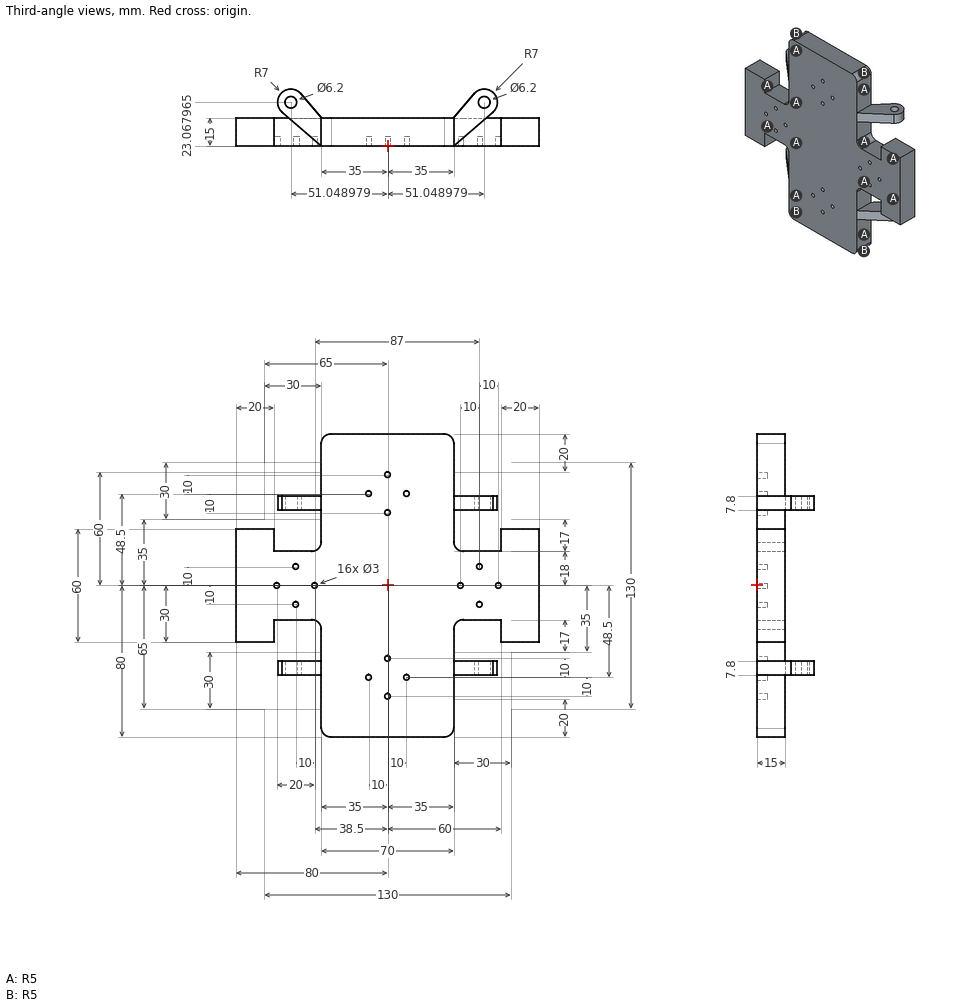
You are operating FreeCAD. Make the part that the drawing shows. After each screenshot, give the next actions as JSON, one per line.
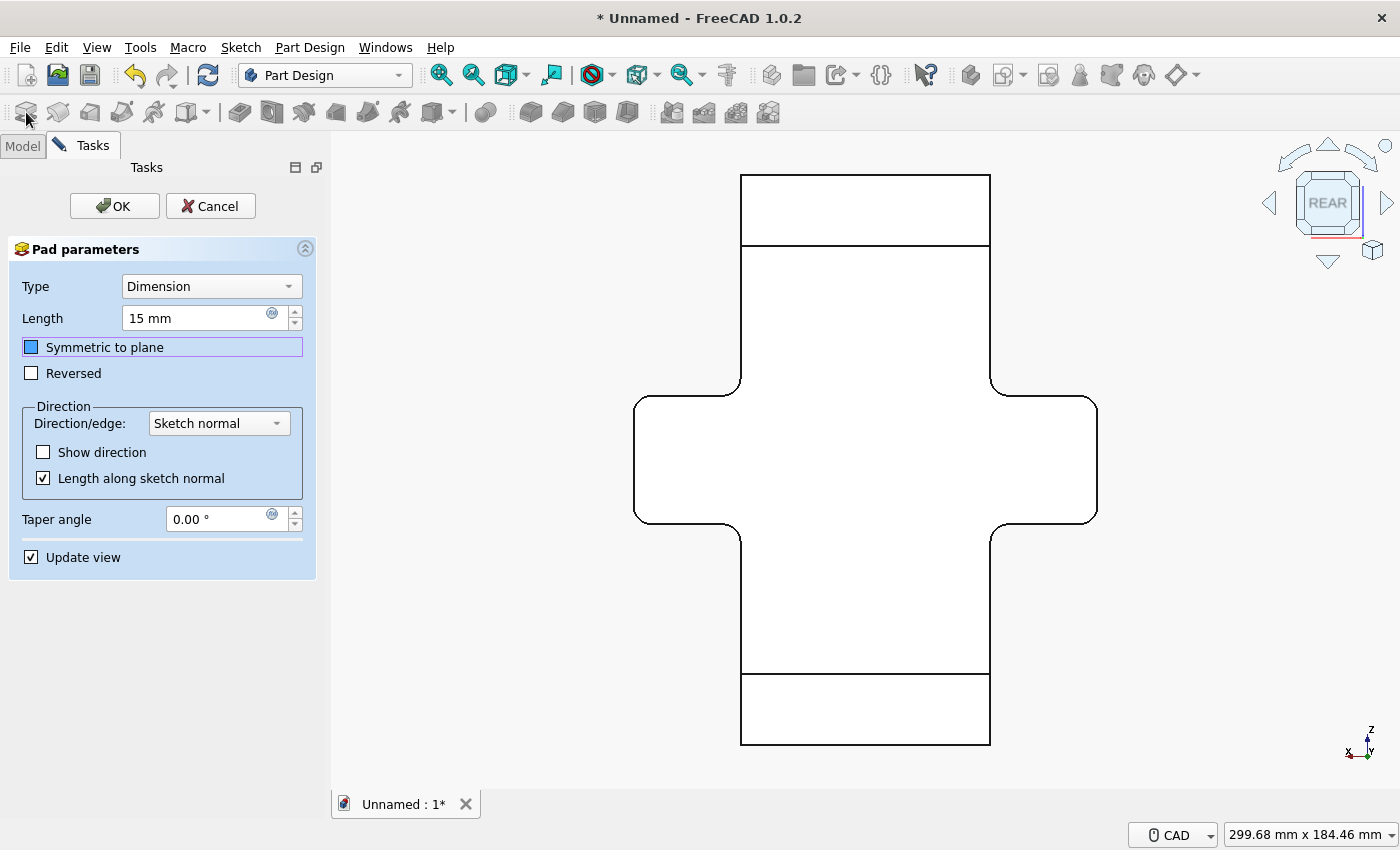
{"action": "left_click", "coordinate": [30, 373]}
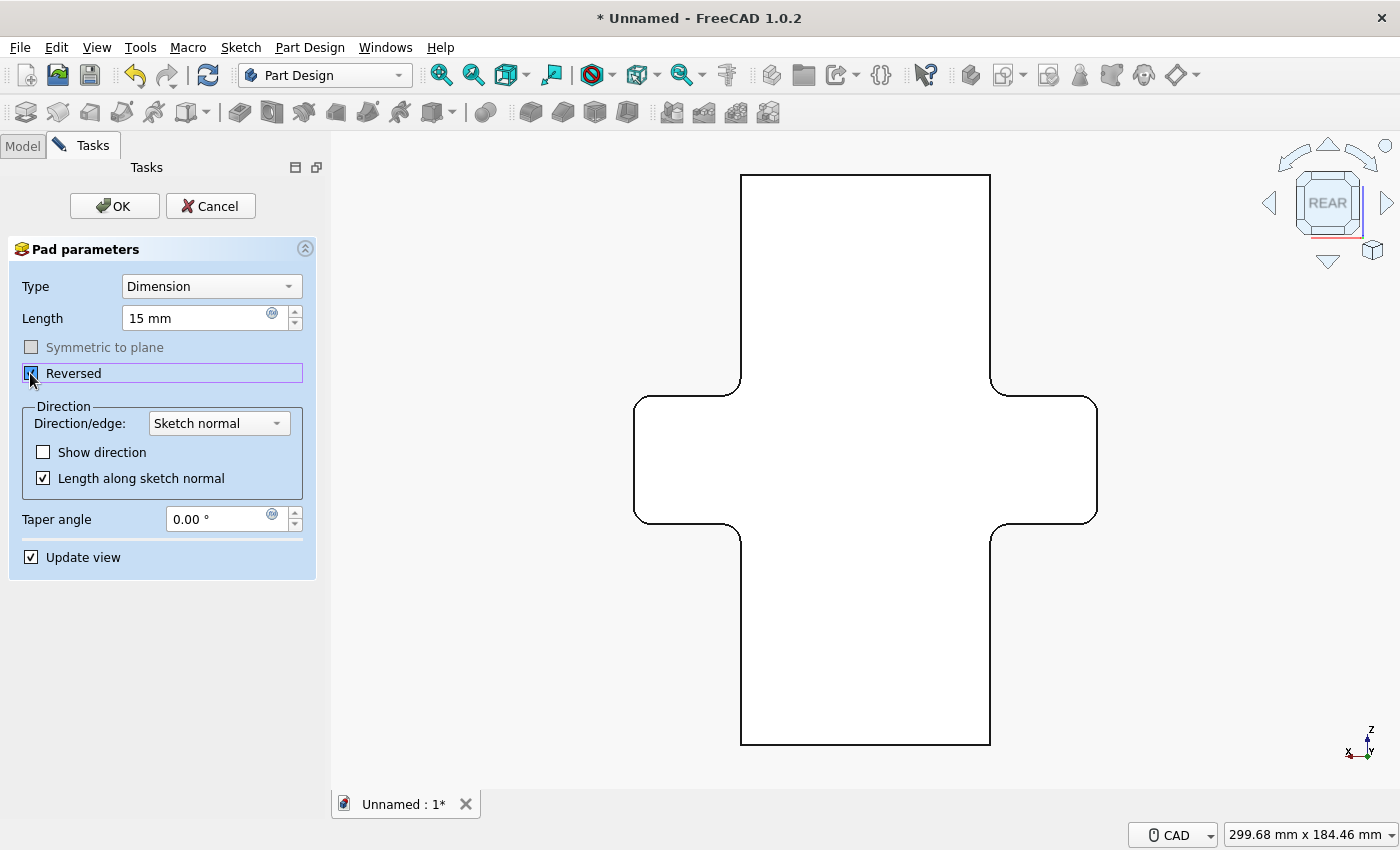
{"action": "left_click", "coordinate": [115, 206]}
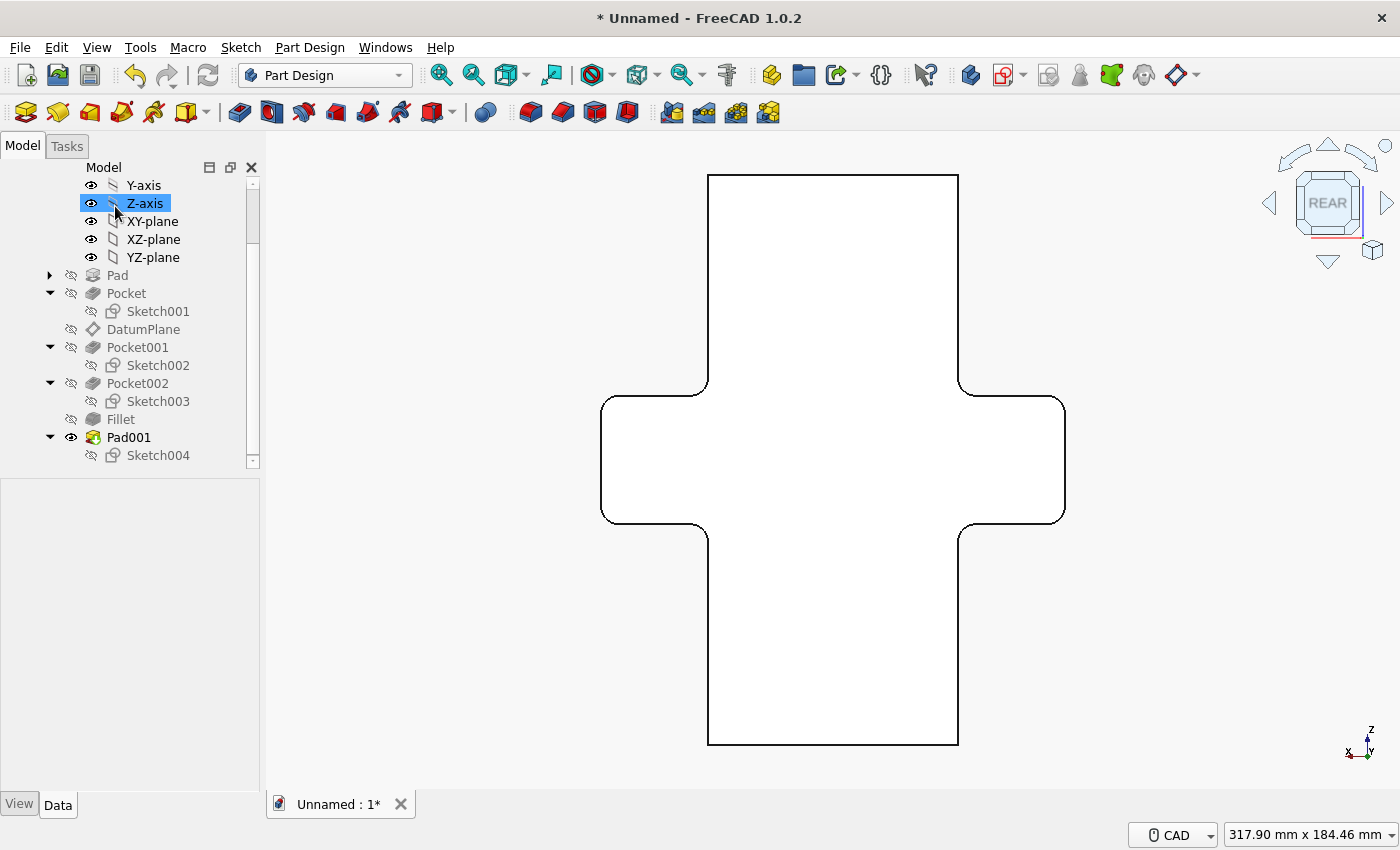
{"action": "scroll", "coordinate": [160, 325], "scroll_direction": "down", "scroll_amount": 3}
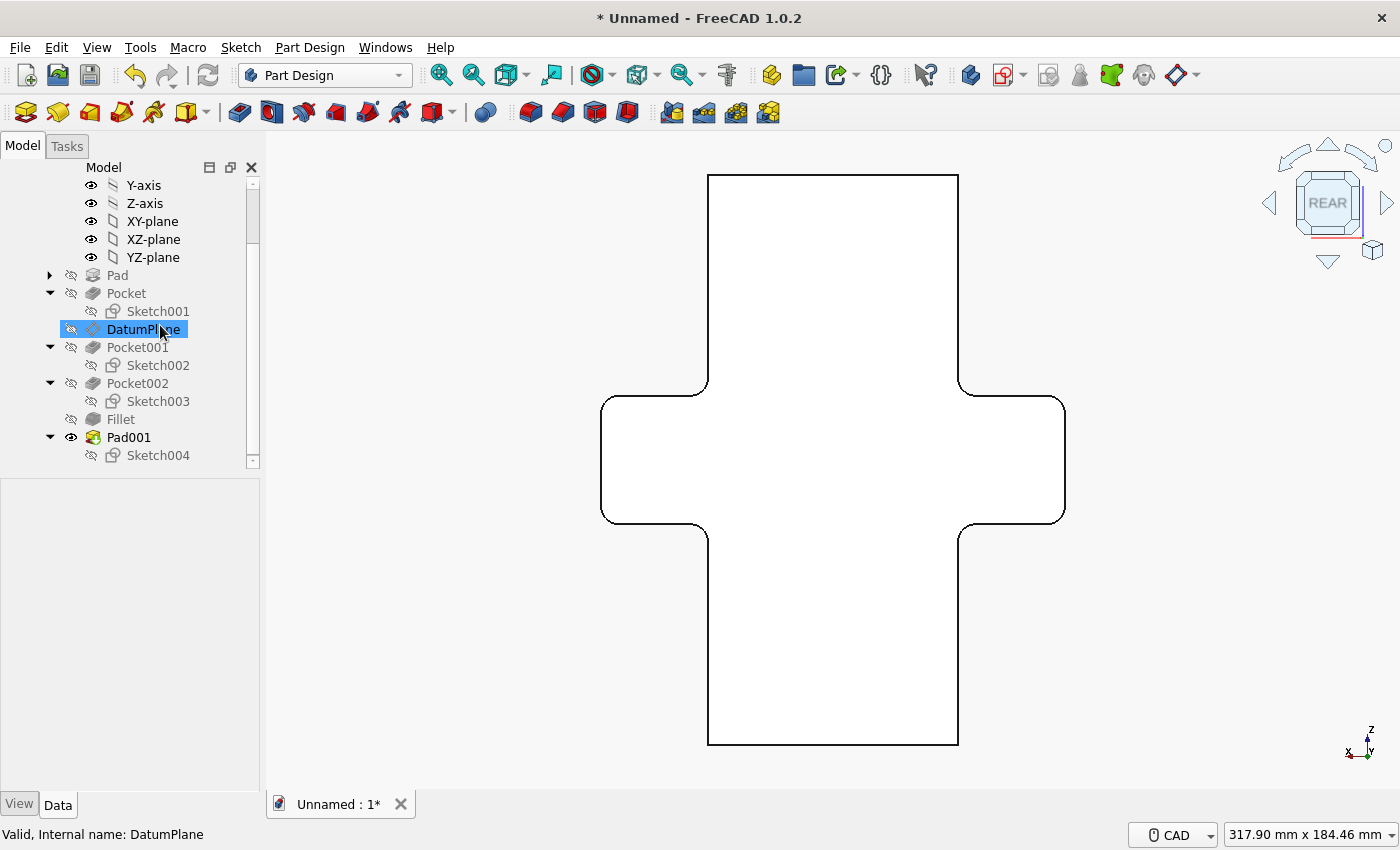
{"action": "scroll", "coordinate": [160, 325], "scroll_direction": "up", "scroll_amount": 15}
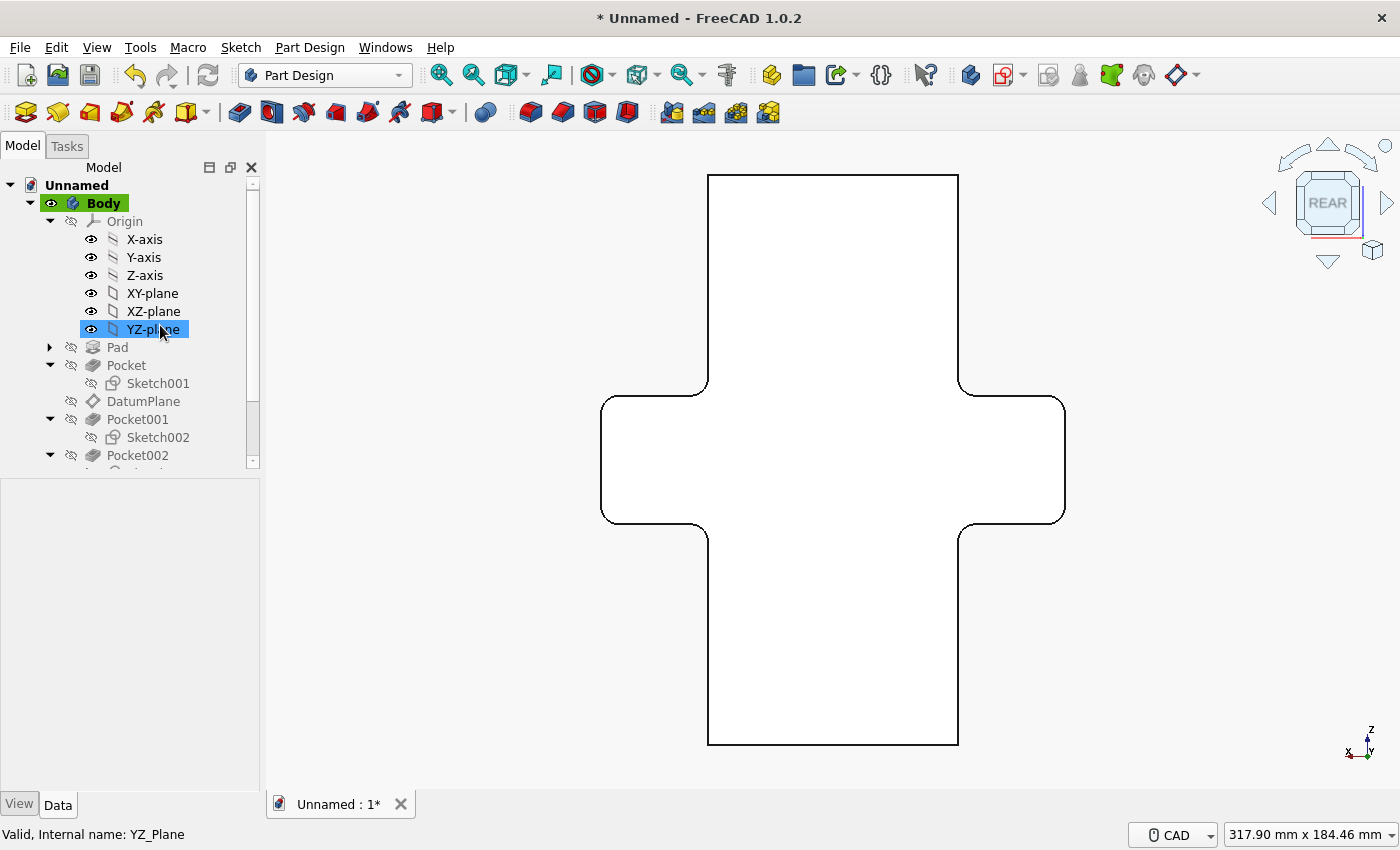
{"action": "left_click", "coordinate": [136, 293]}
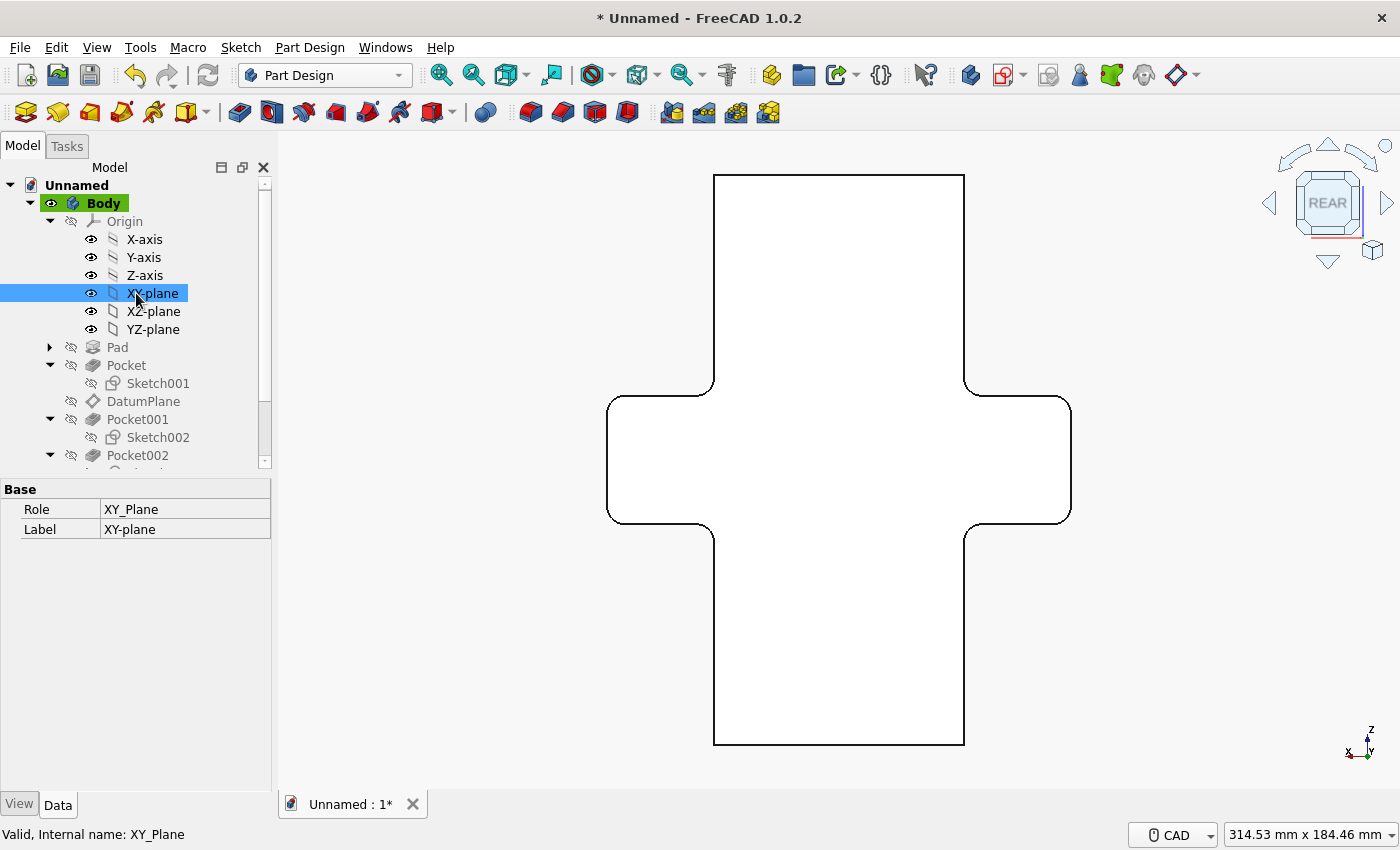
{"action": "left_click", "coordinate": [1176, 76]}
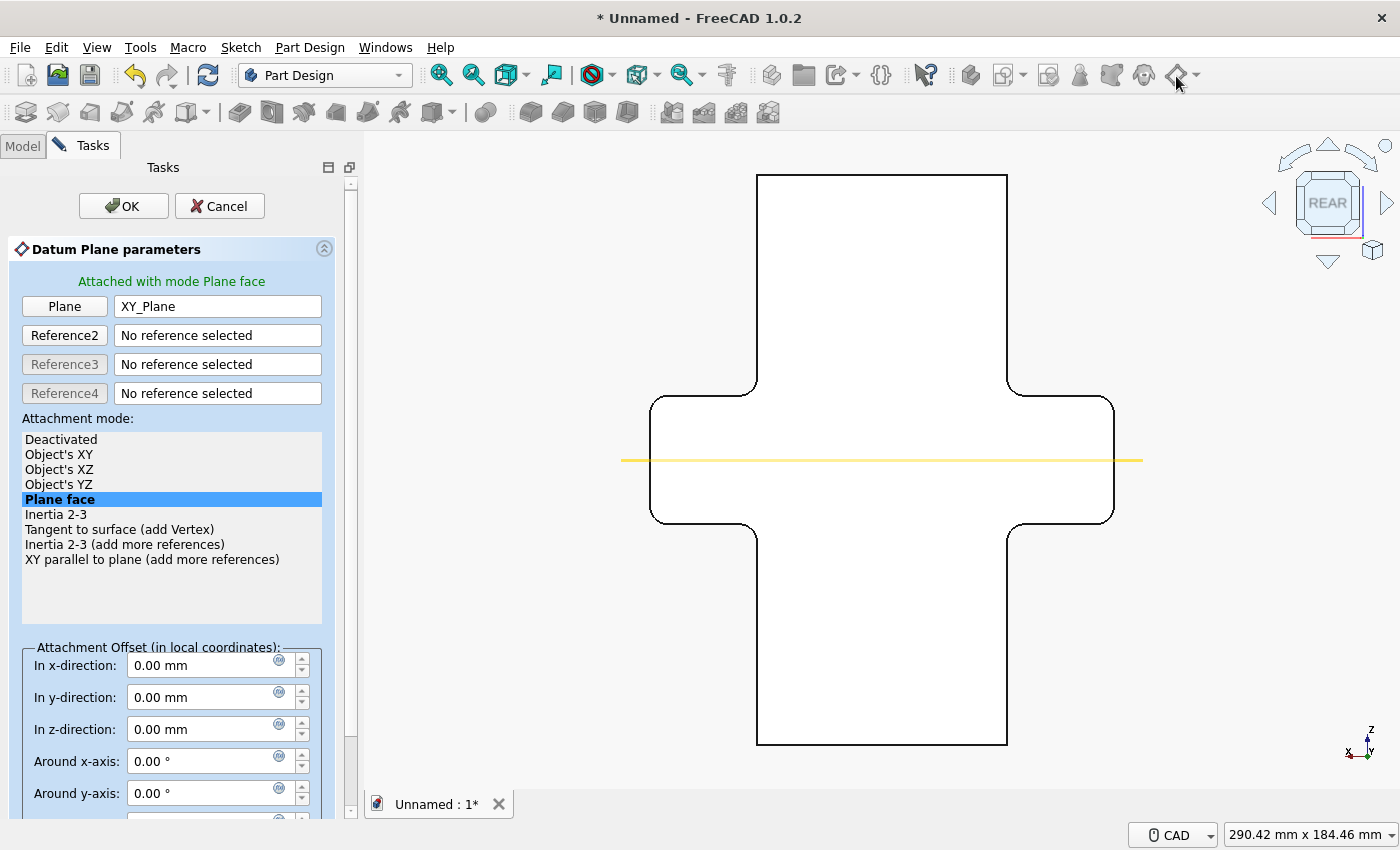
{"action": "triple_click", "coordinate": [210, 729]}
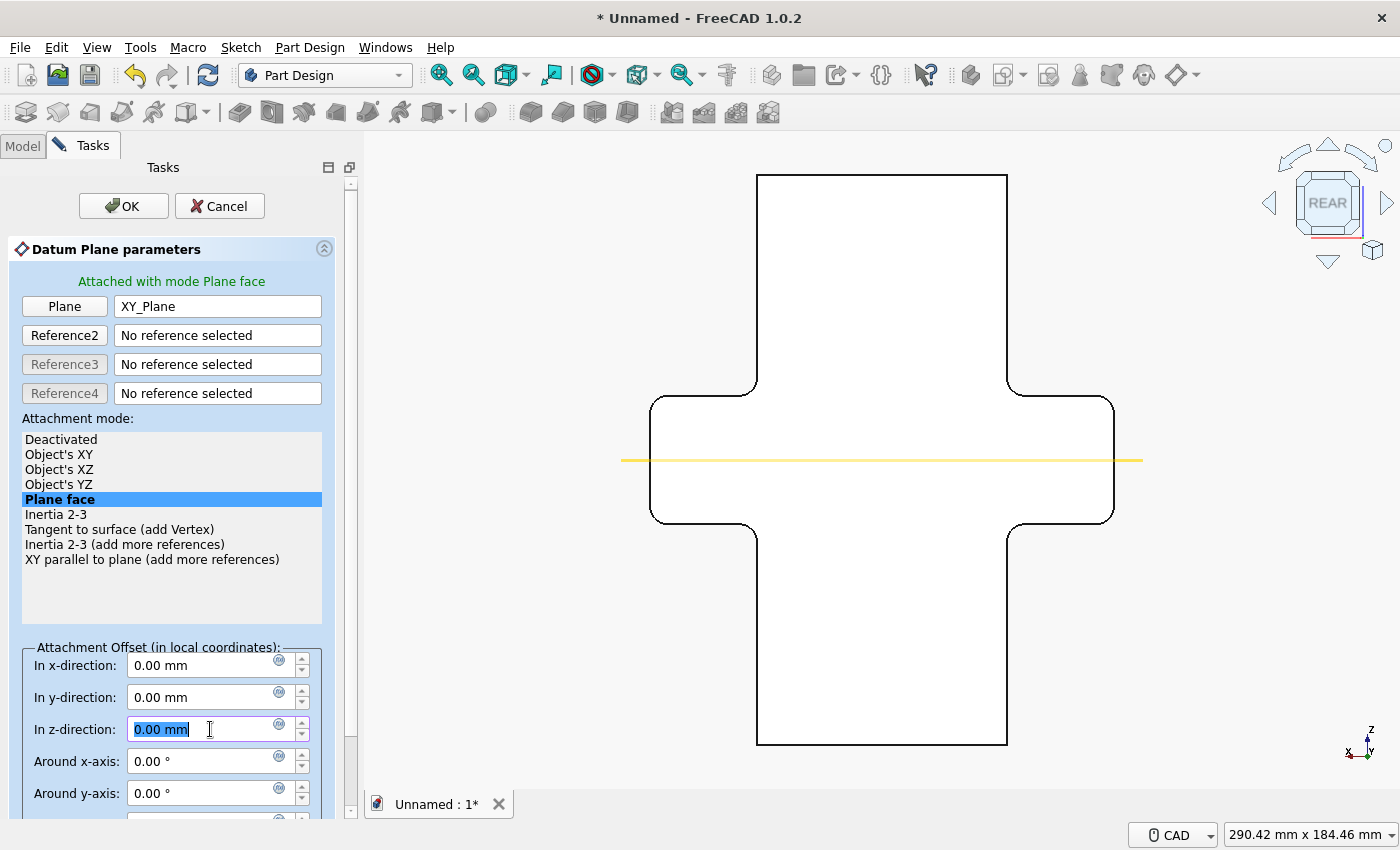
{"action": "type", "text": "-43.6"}
{"action": "key", "text": "Tab"}